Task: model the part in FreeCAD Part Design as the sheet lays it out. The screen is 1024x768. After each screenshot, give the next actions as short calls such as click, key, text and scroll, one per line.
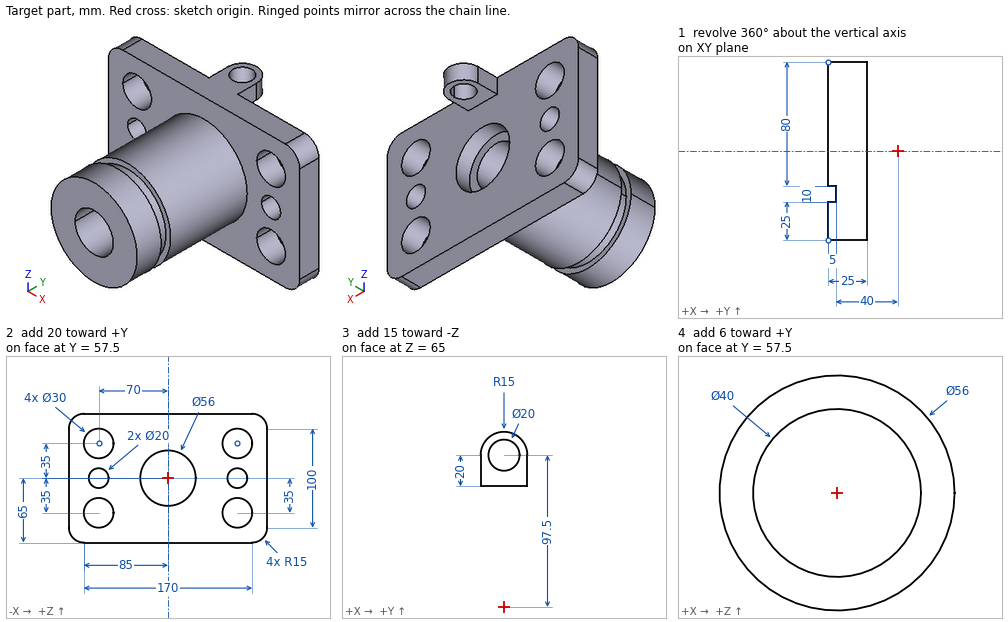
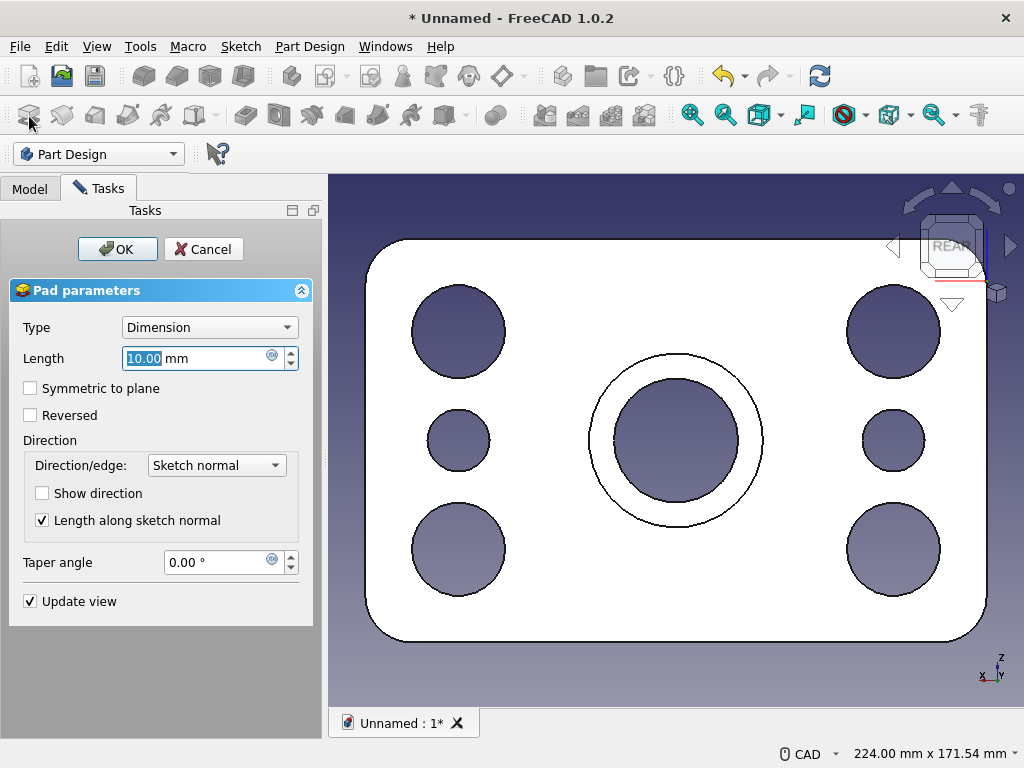
text(20)
key(Tab)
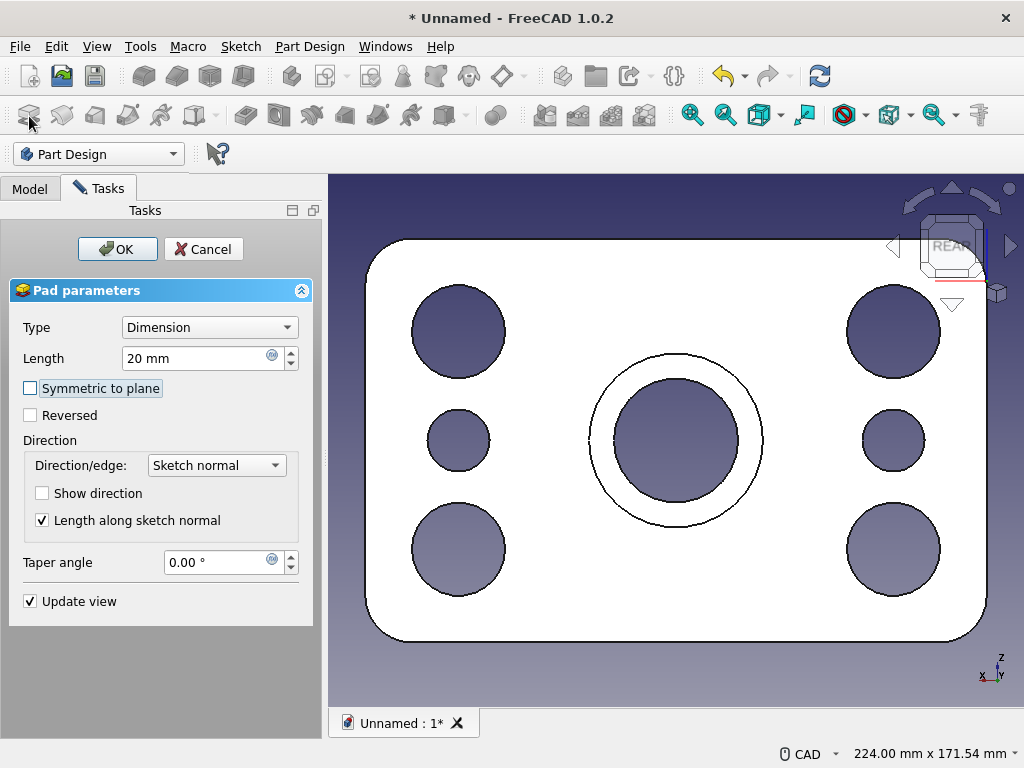
click(118, 249)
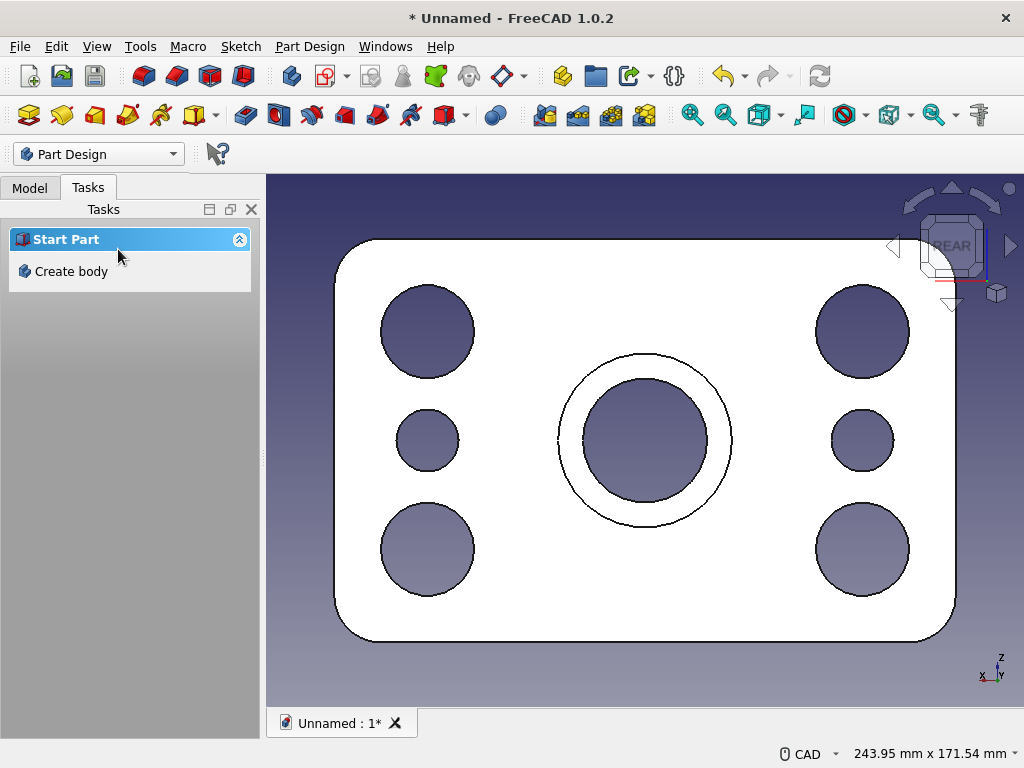
key(0)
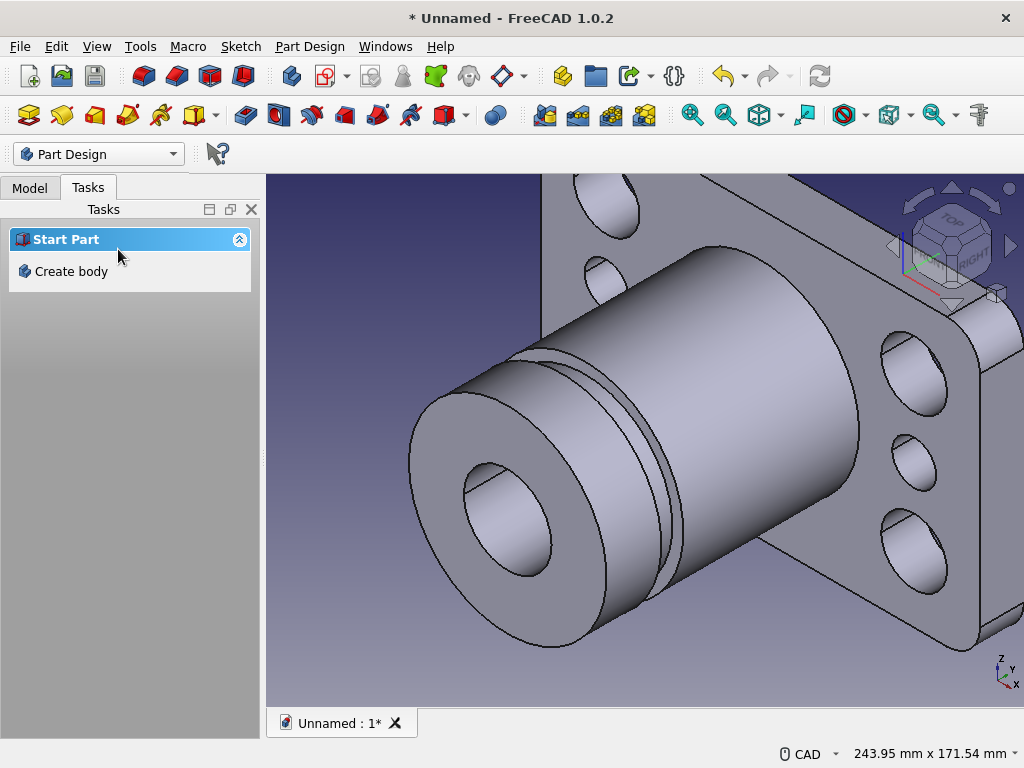
click(693, 116)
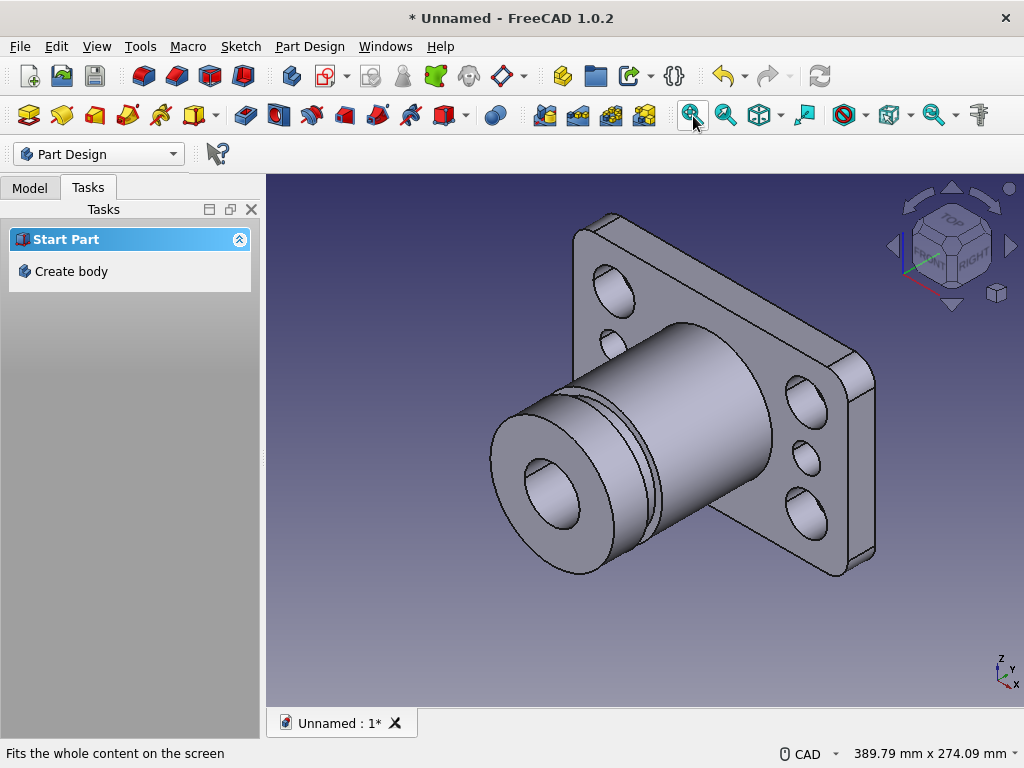
click(824, 348)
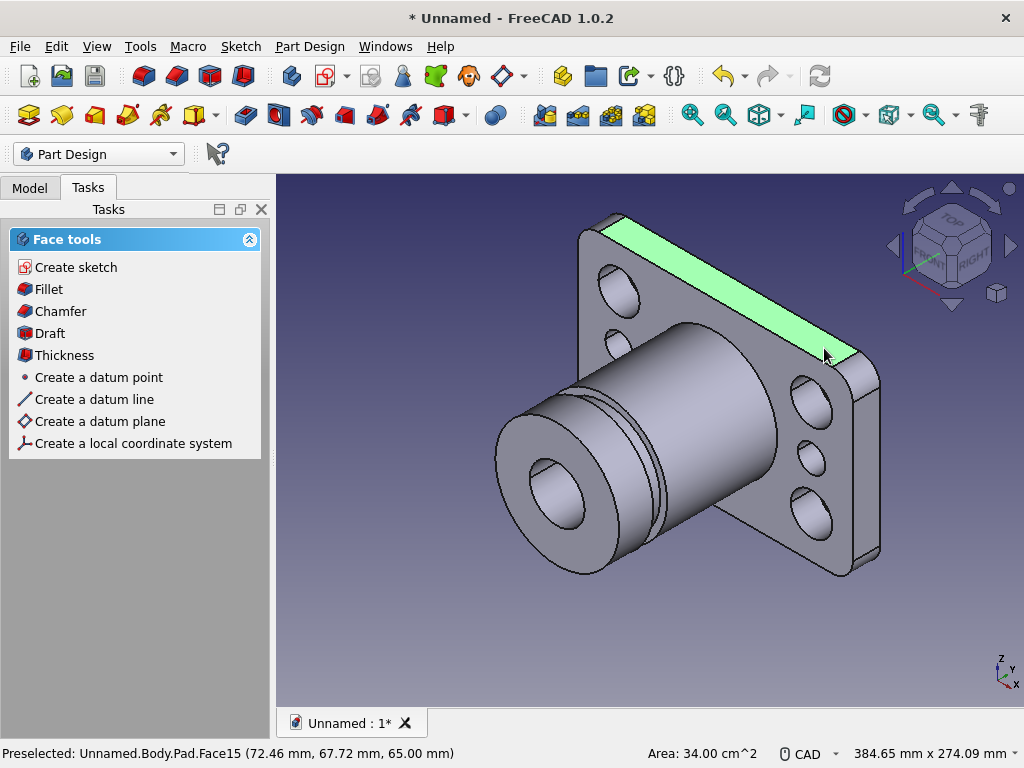
click(324, 76)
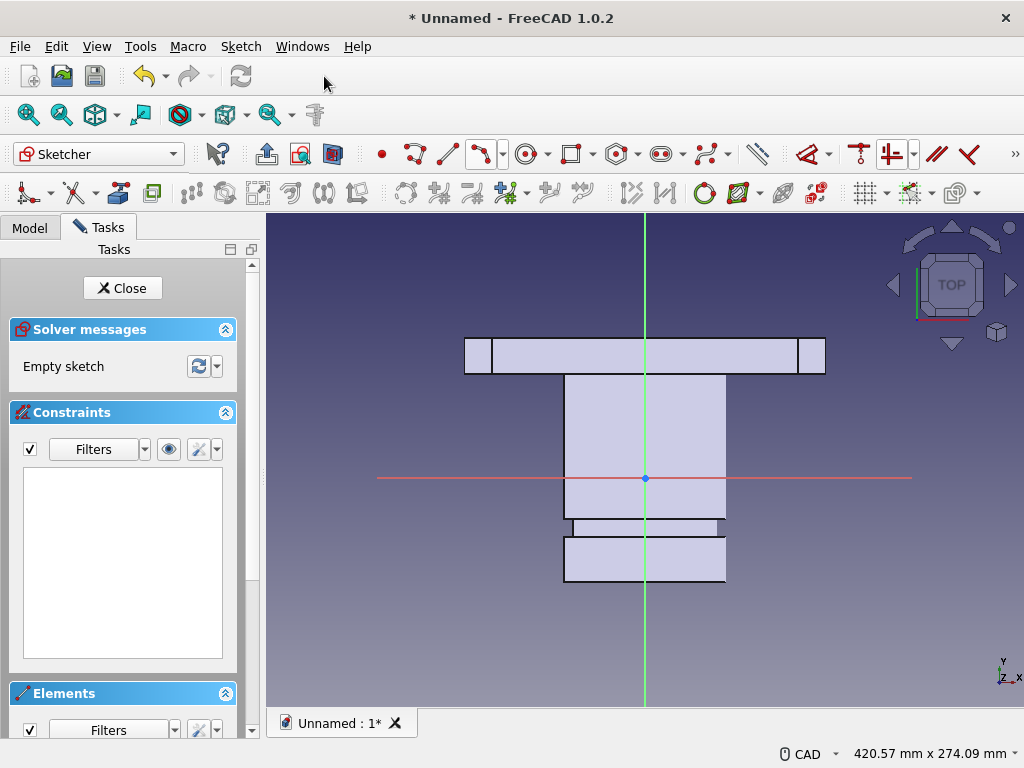
scroll(662, 268, up, 8)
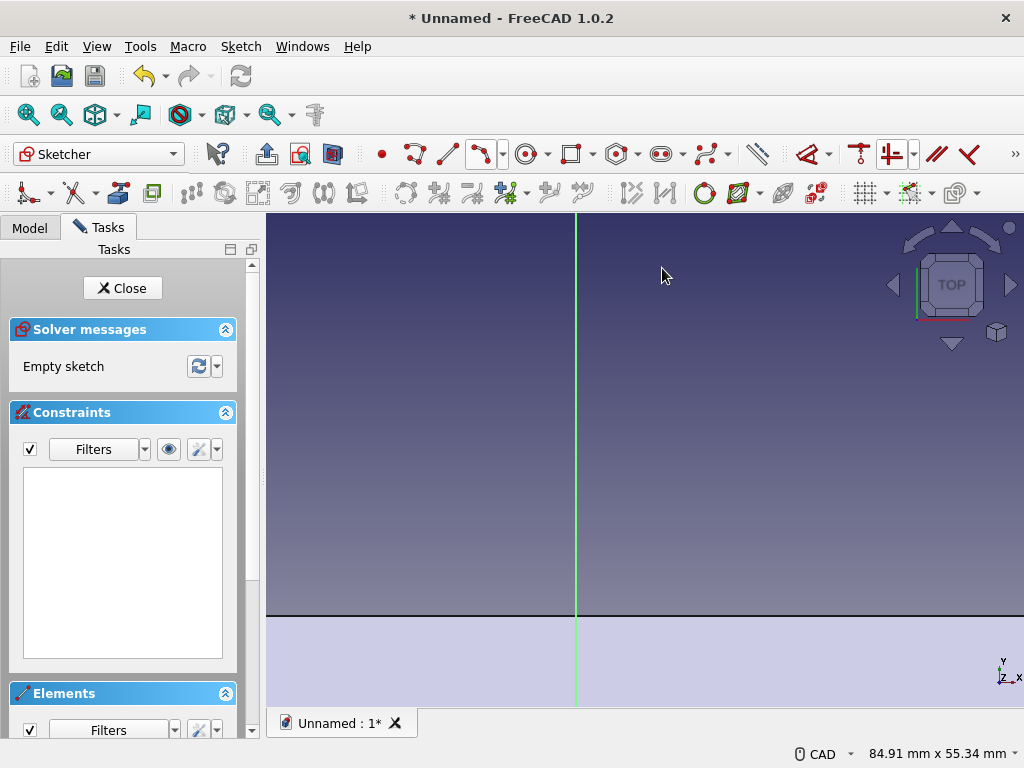
click(415, 154)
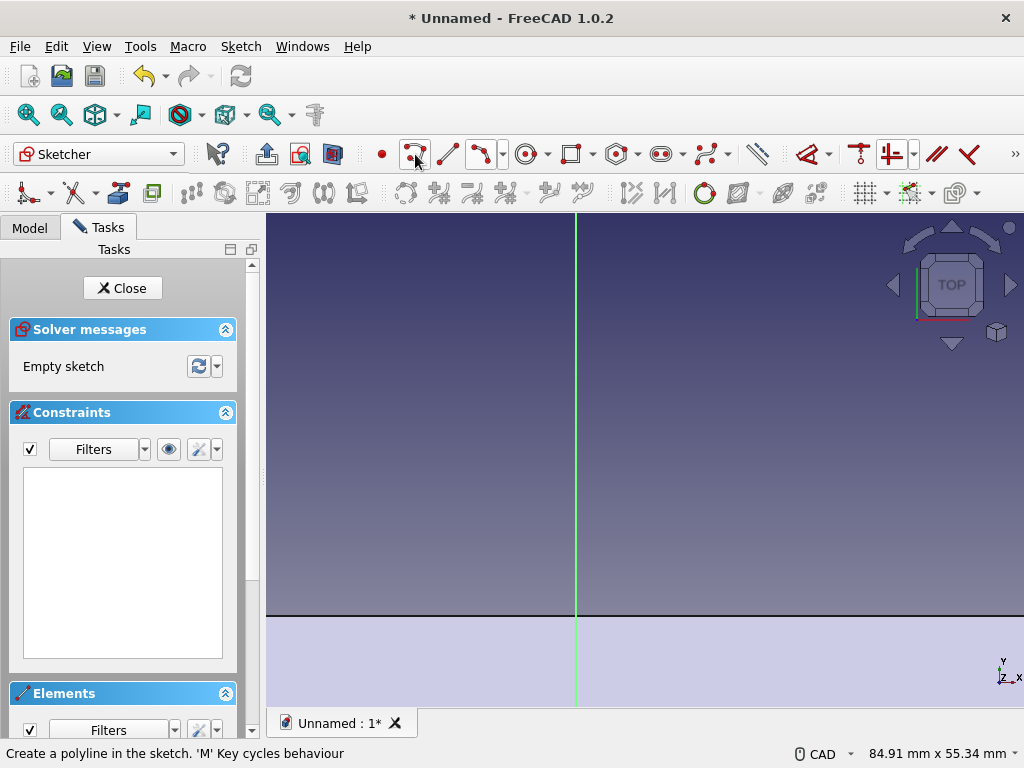
click(442, 437)
click(442, 616)
click(710, 616)
click(710, 437)
right_click(710, 437)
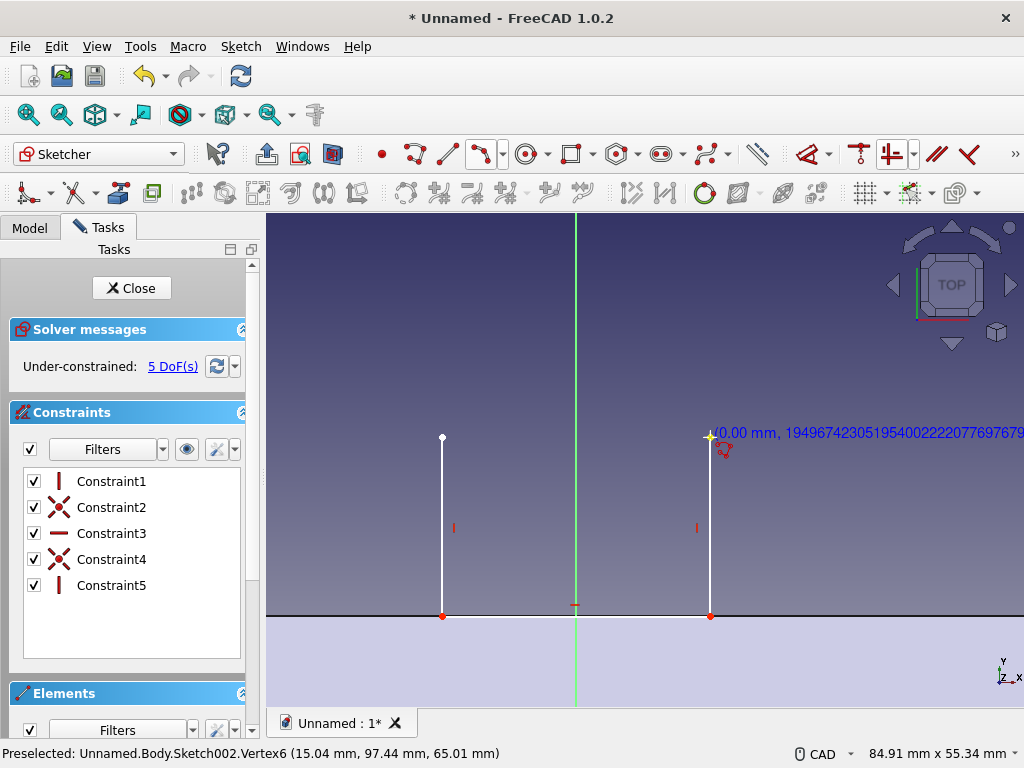
click(480, 154)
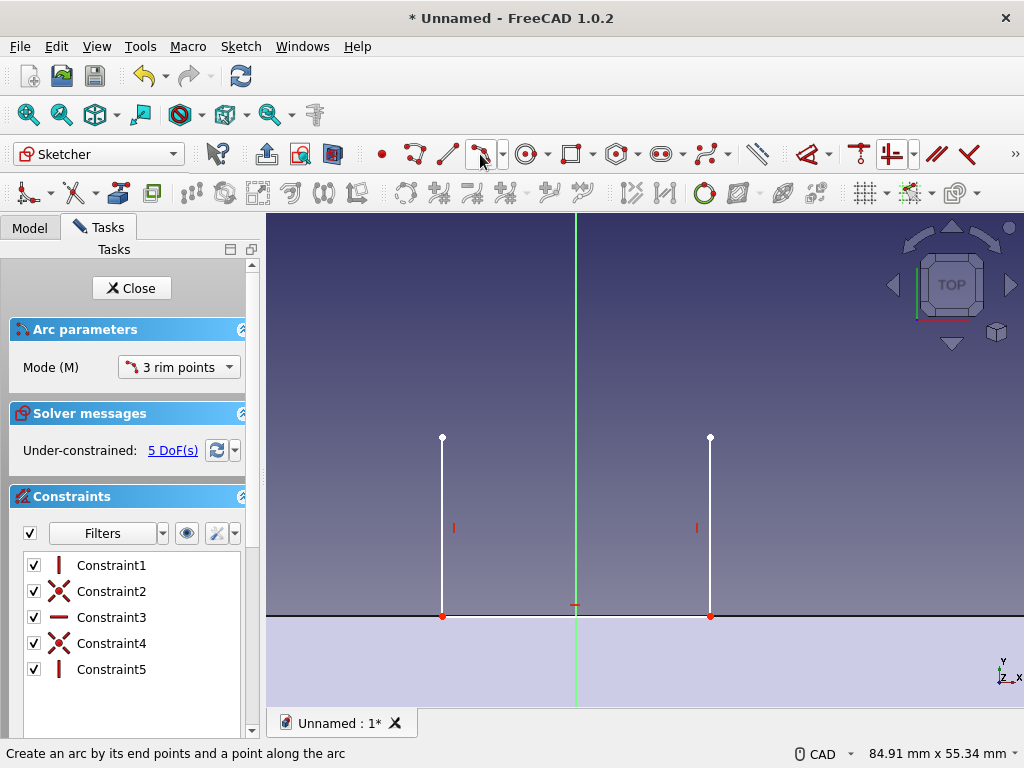
click(710, 438)
click(442, 438)
click(617, 310)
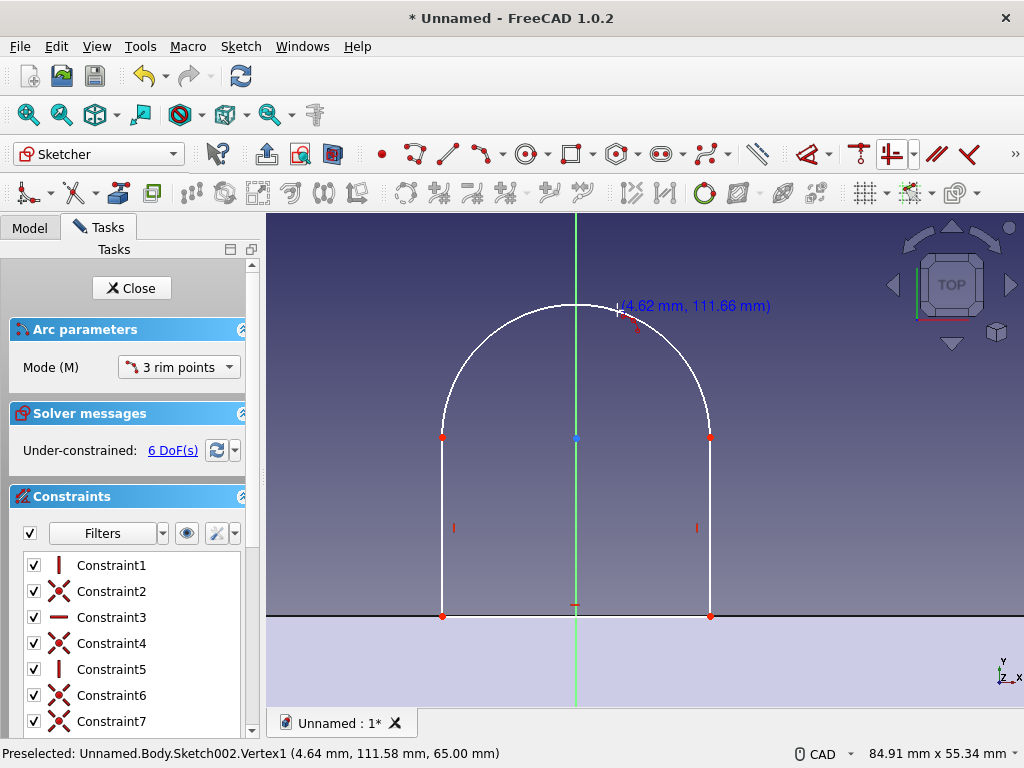
click(526, 154)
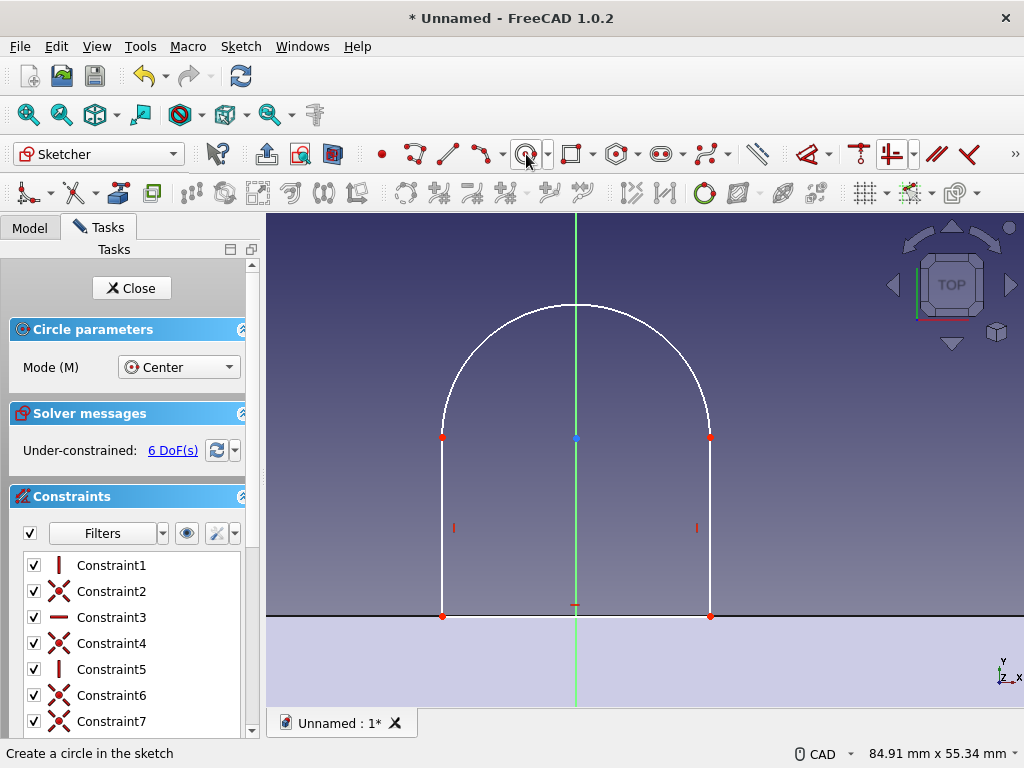
click(576, 437)
move(639, 374)